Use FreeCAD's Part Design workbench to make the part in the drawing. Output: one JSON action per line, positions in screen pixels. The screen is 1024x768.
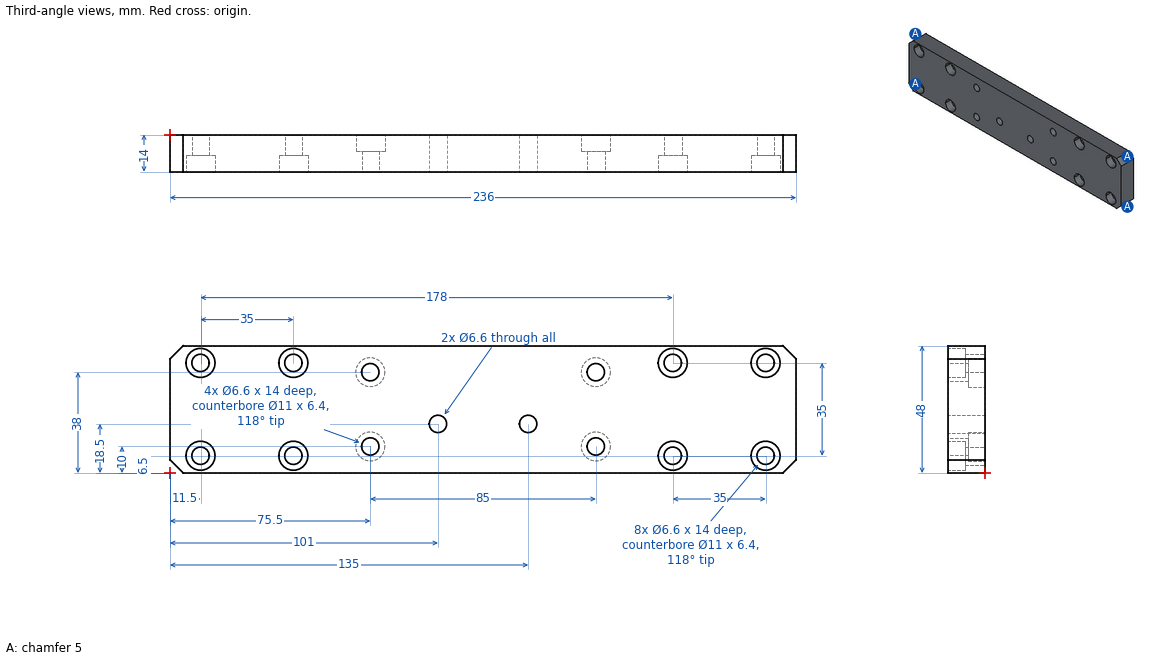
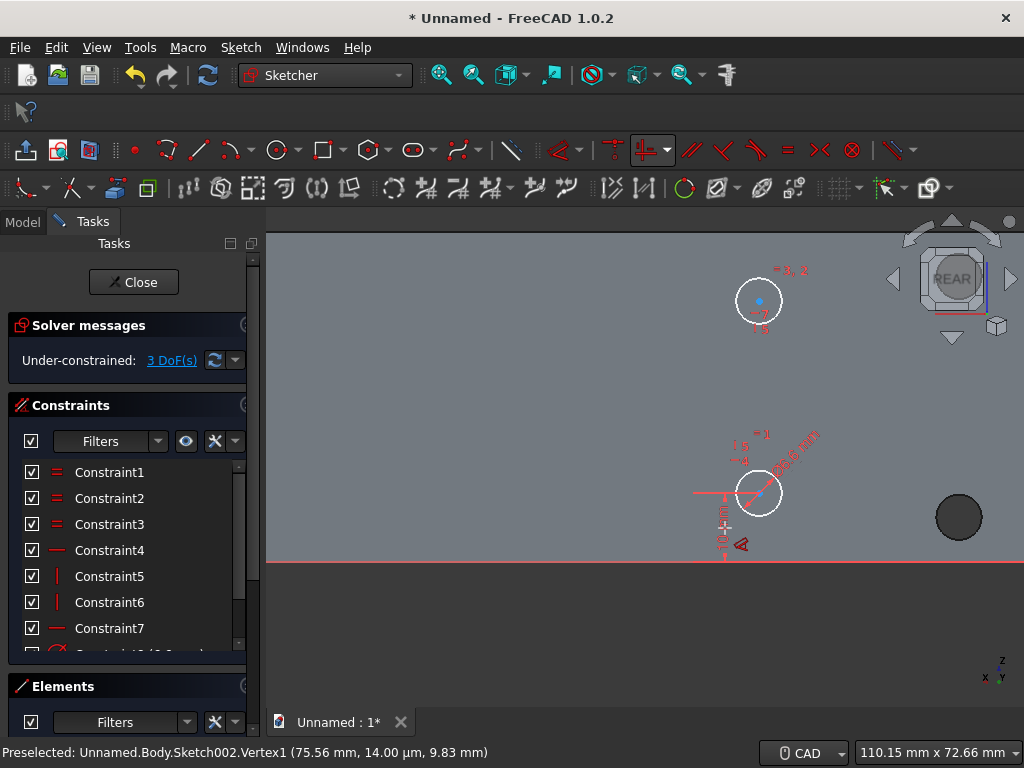
{"action": "left_click", "coordinate": [759, 301]}
{"action": "left_click", "coordinate": [725, 432]}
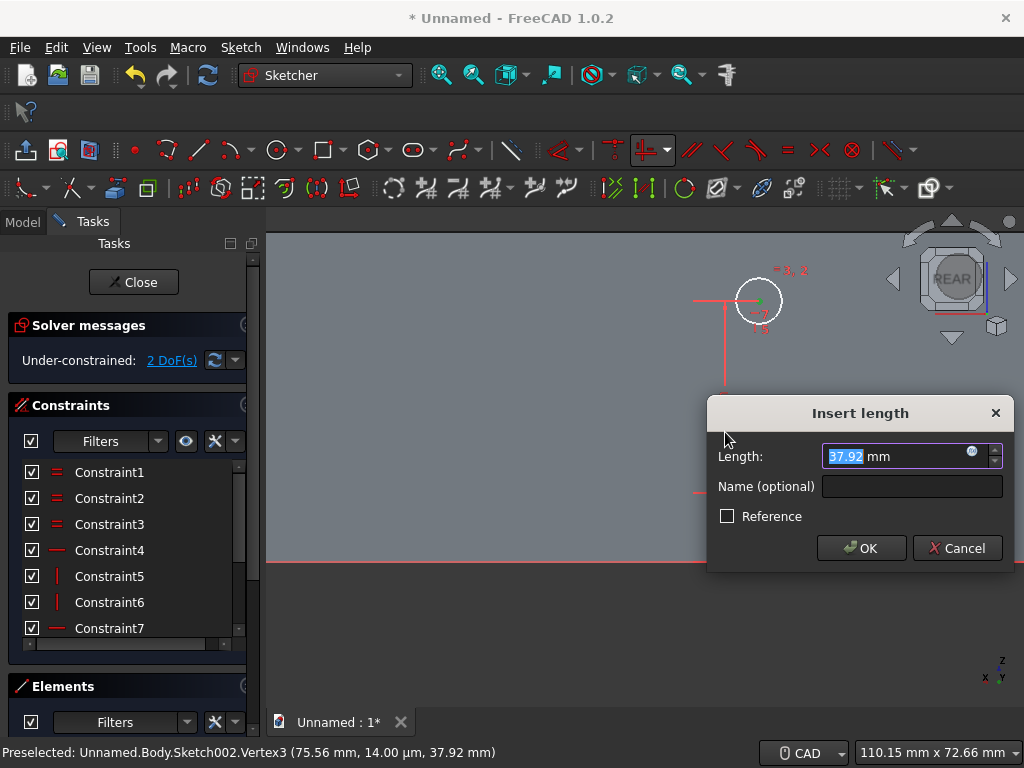
{"action": "type", "text": "38"}
{"action": "key", "text": "Return"}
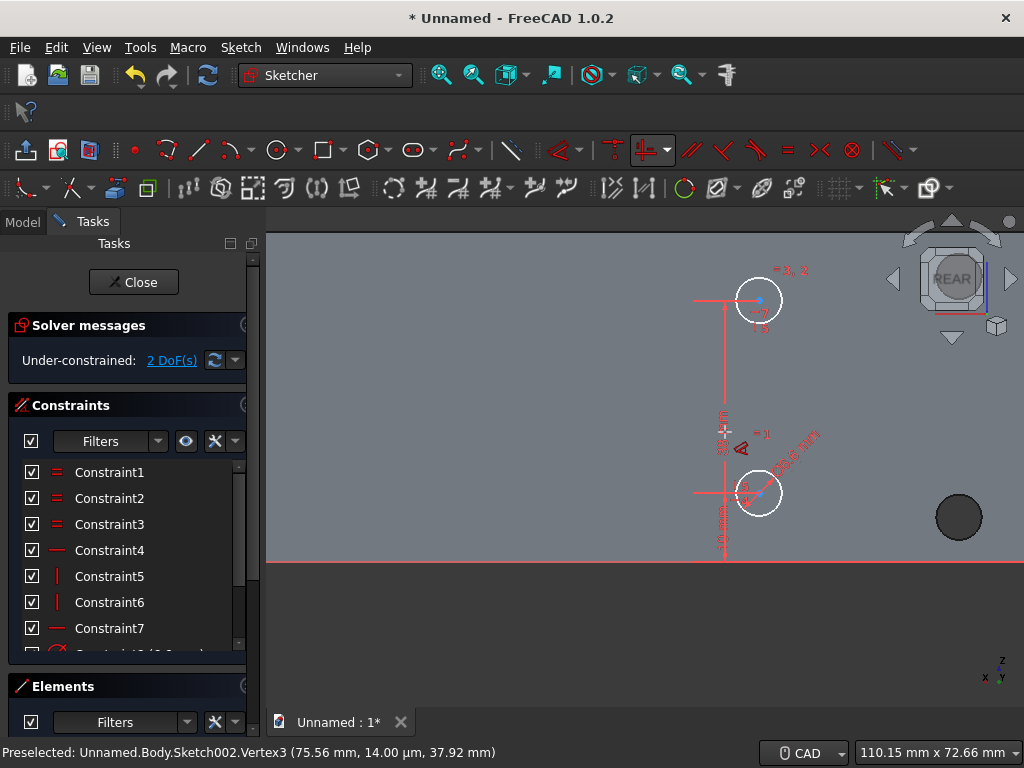
{"action": "left_click", "coordinate": [759, 493]}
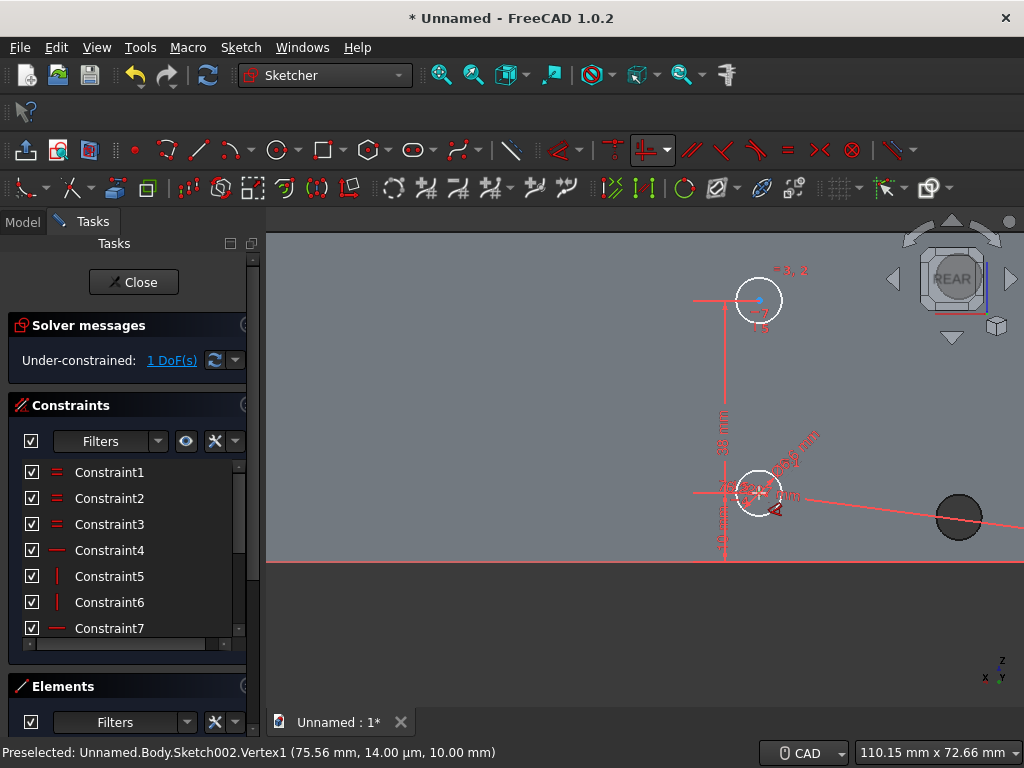
{"action": "scroll", "coordinate": [496, 479], "scroll_direction": "down", "scroll_amount": 5}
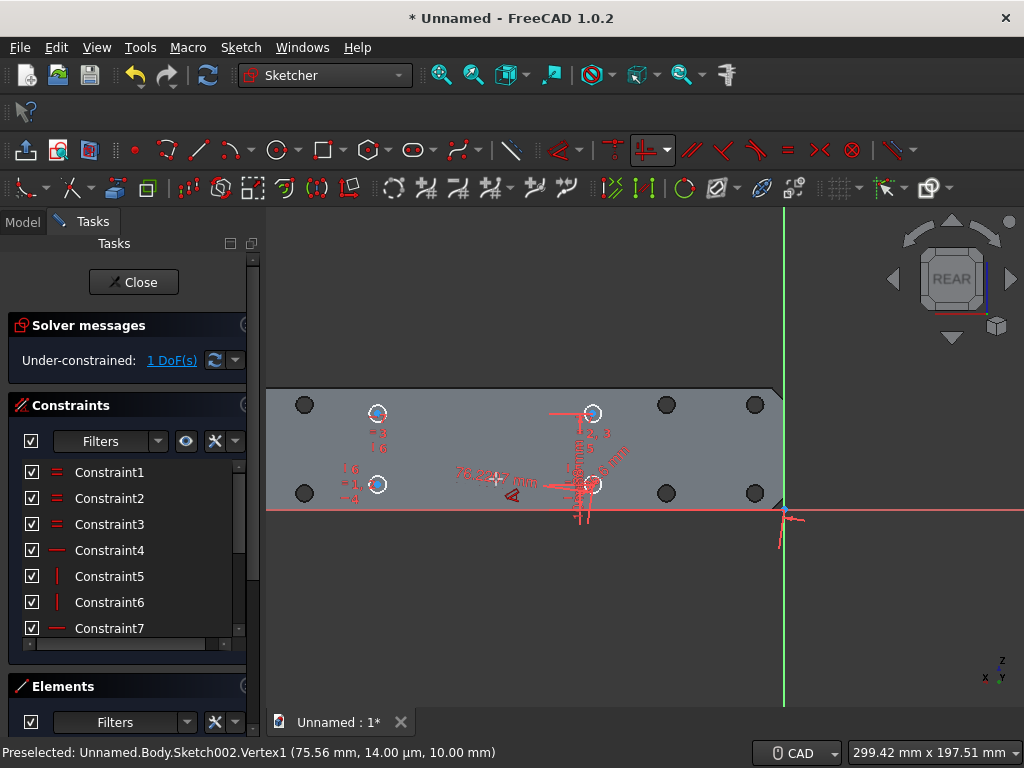
{"action": "left_click", "coordinate": [378, 485]}
{"action": "left_click", "coordinate": [485, 451]}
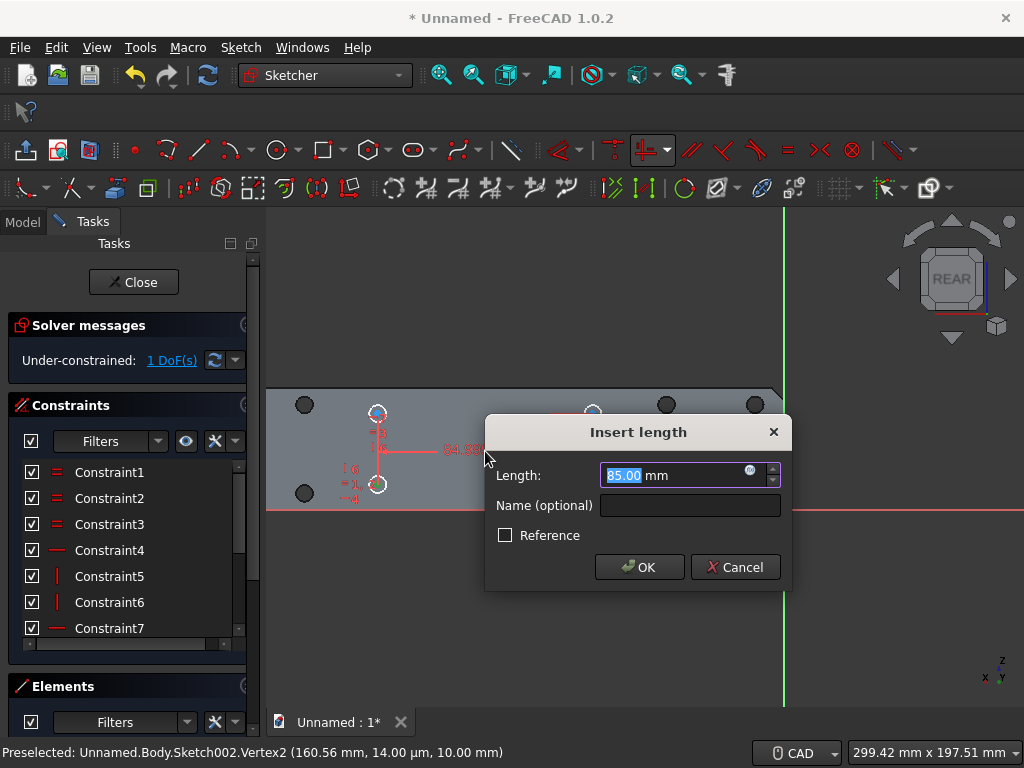
{"action": "type", "text": "85"}
{"action": "key", "text": "Return"}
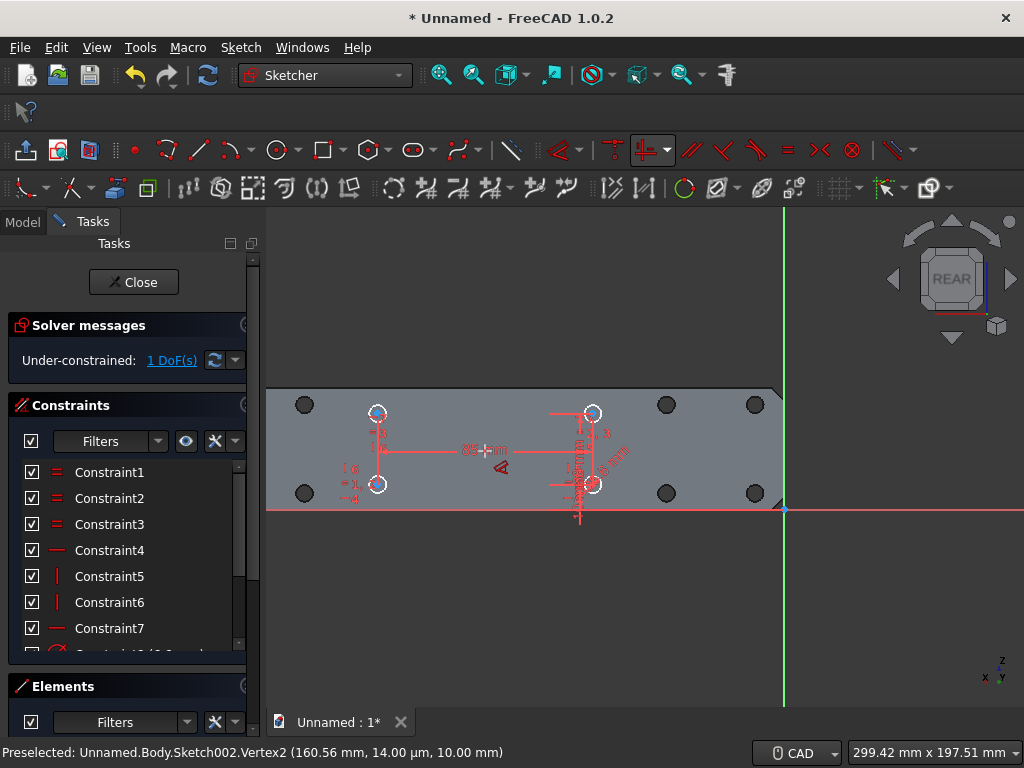
{"action": "left_click", "coordinate": [593, 485]}
{"action": "left_click", "coordinate": [689, 544]}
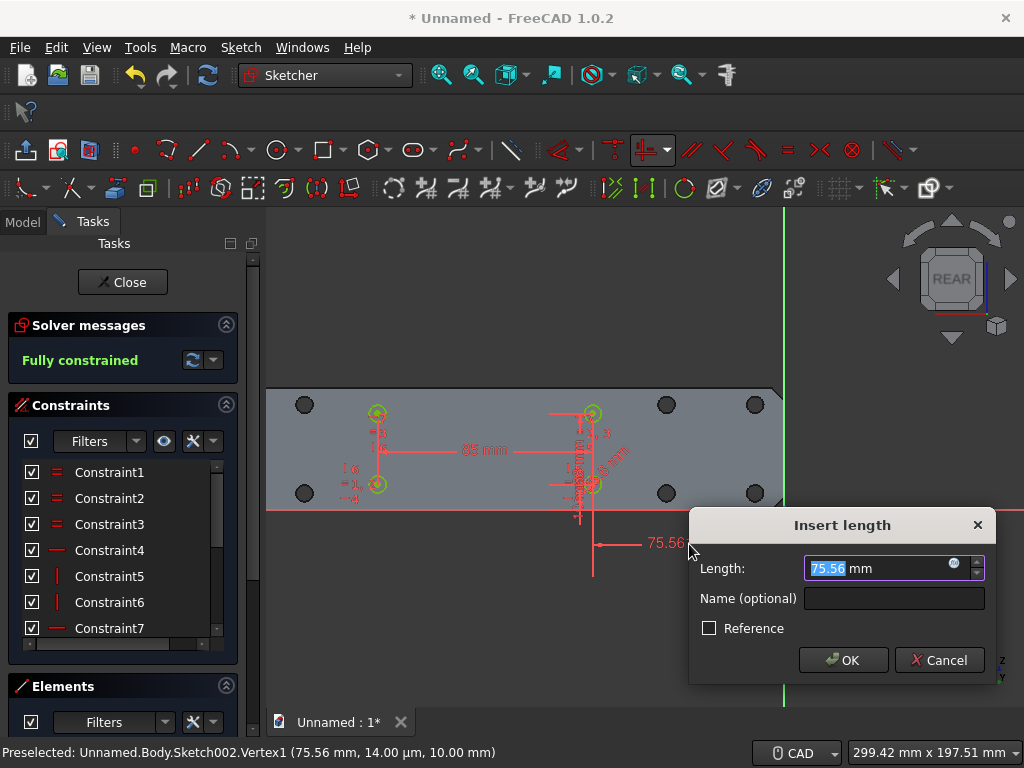
{"action": "type", "text": "75.5"}
{"action": "key", "text": "Return"}
{"action": "key", "text": "Escape"}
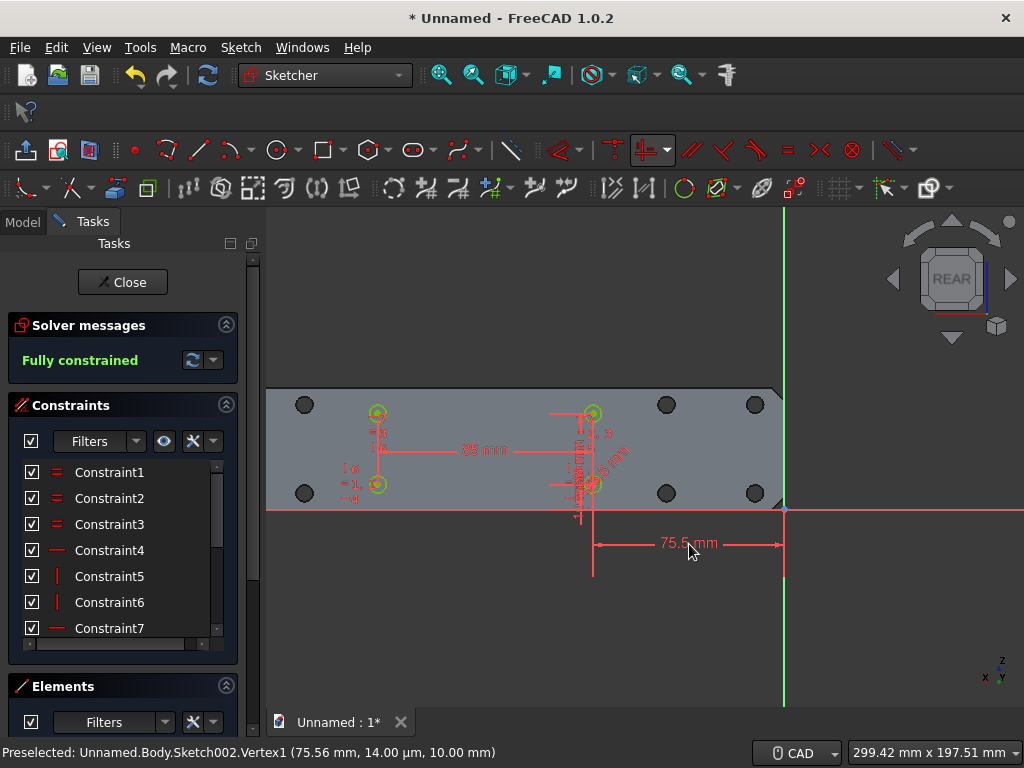
{"action": "left_click", "coordinate": [123, 282]}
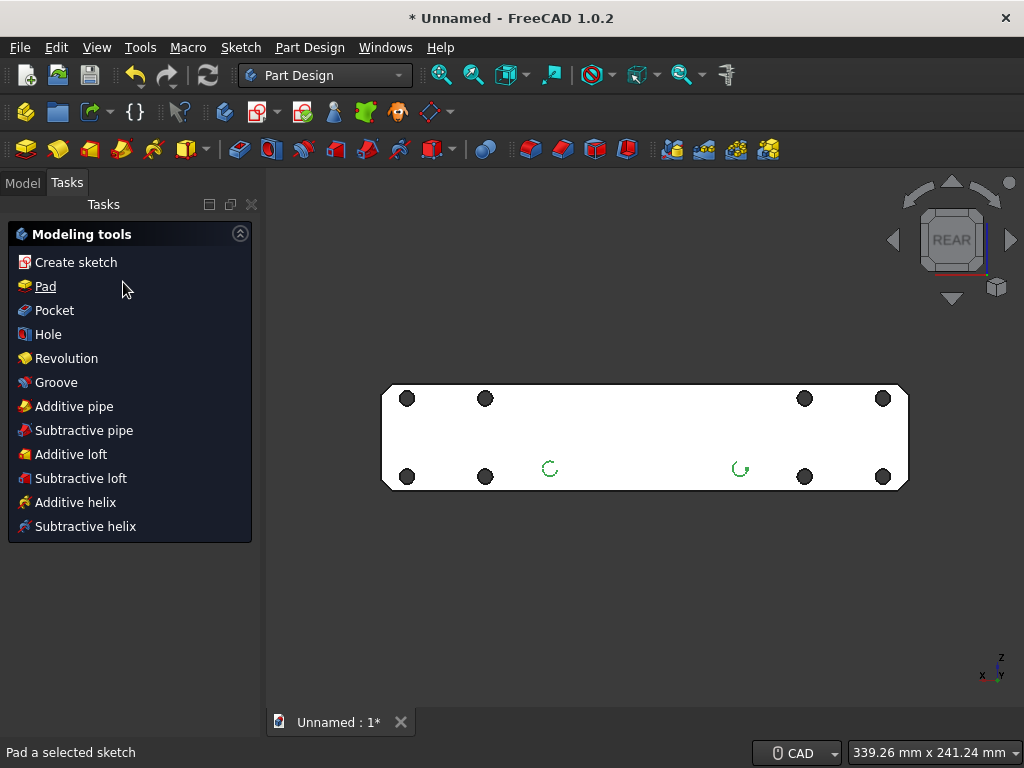
{"action": "left_click", "coordinate": [272, 150]}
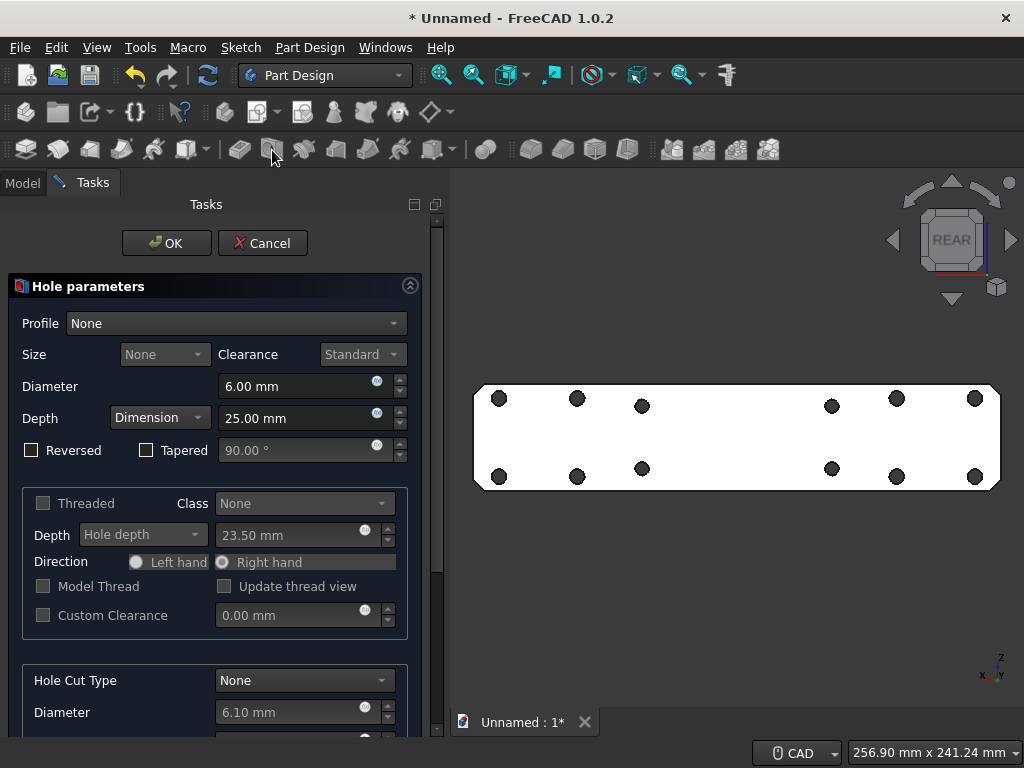
{"action": "triple_click", "coordinate": [305, 386]}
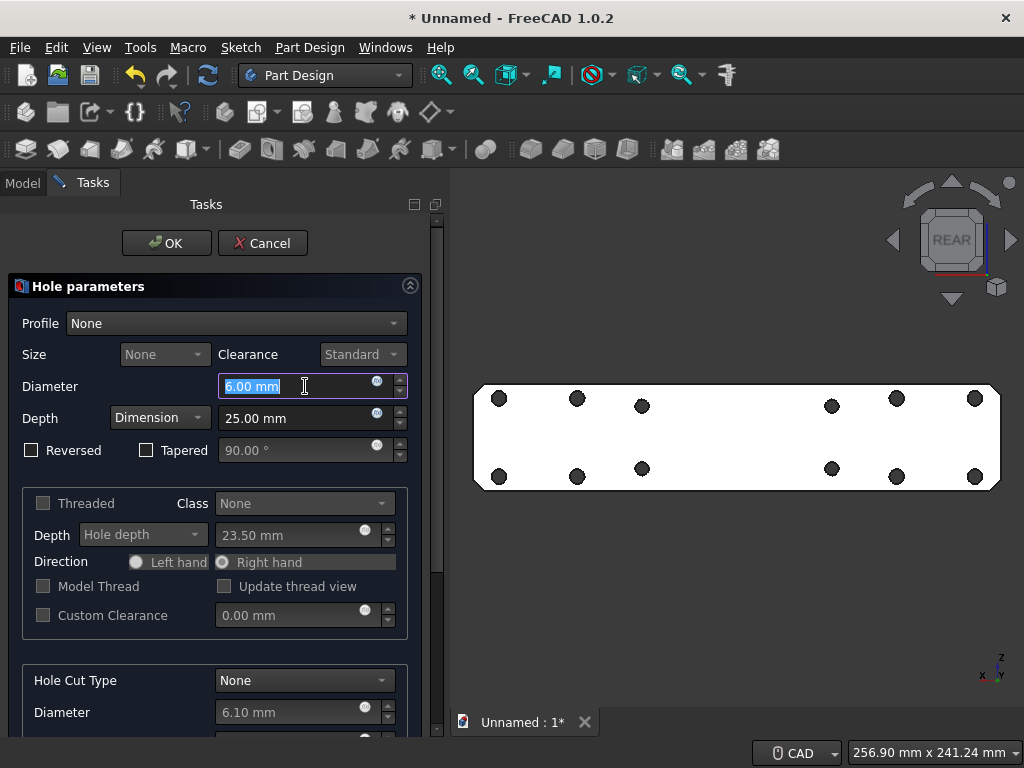
{"action": "type", "text": "6.6"}
{"action": "key", "text": "Tab"}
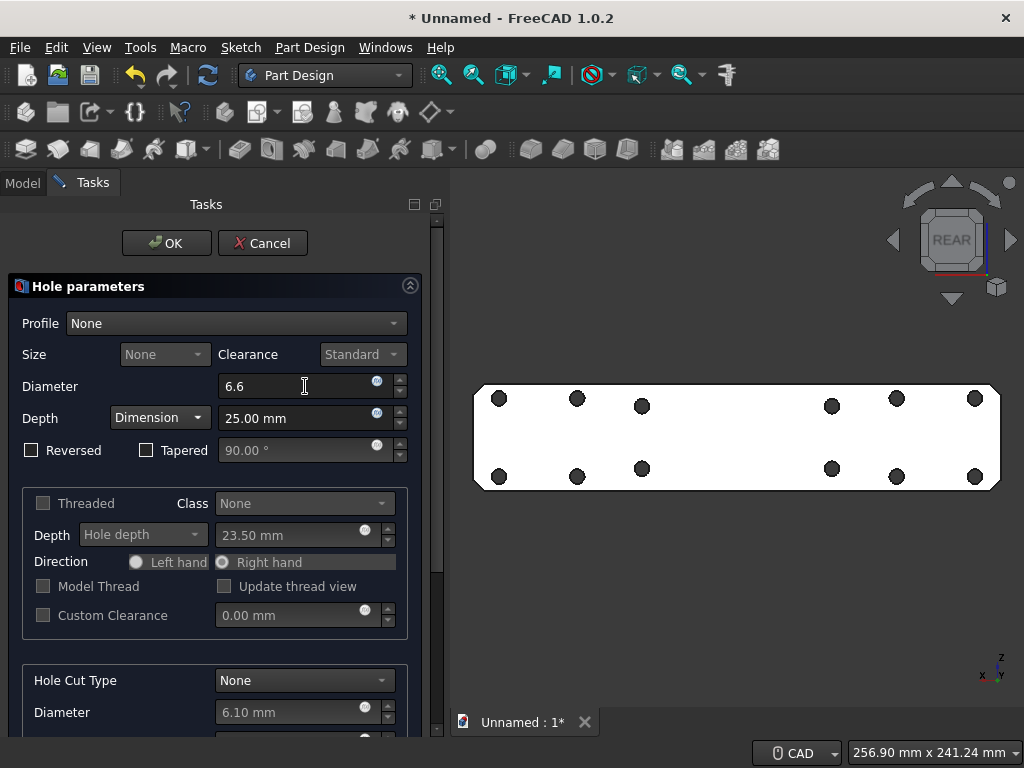
{"action": "triple_click", "coordinate": [305, 418]}